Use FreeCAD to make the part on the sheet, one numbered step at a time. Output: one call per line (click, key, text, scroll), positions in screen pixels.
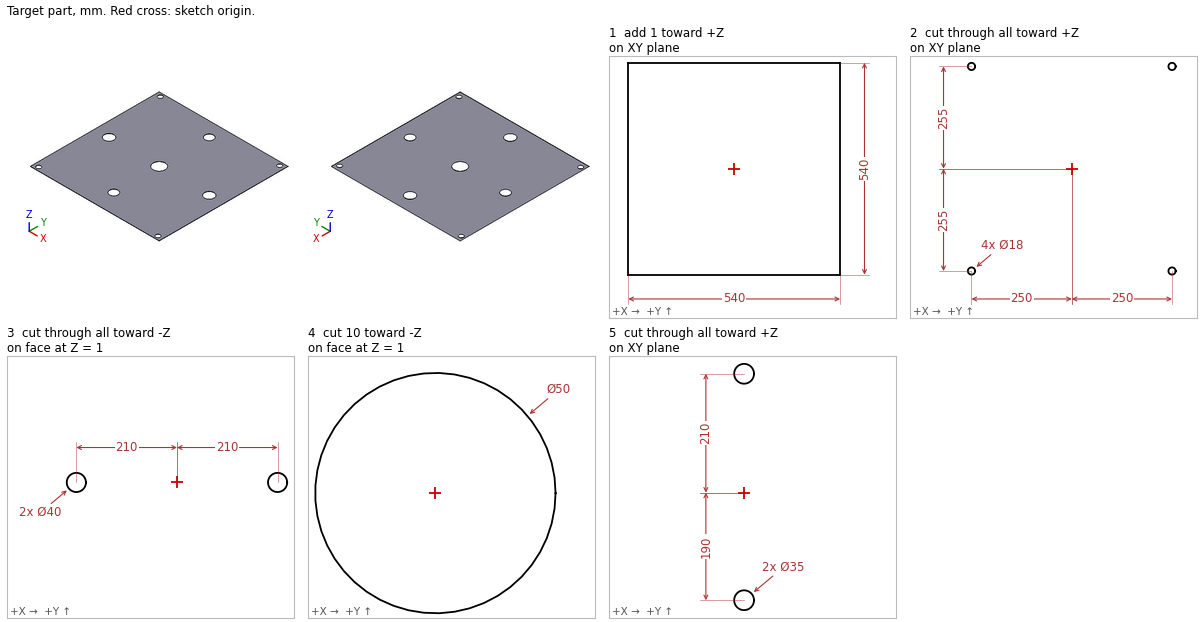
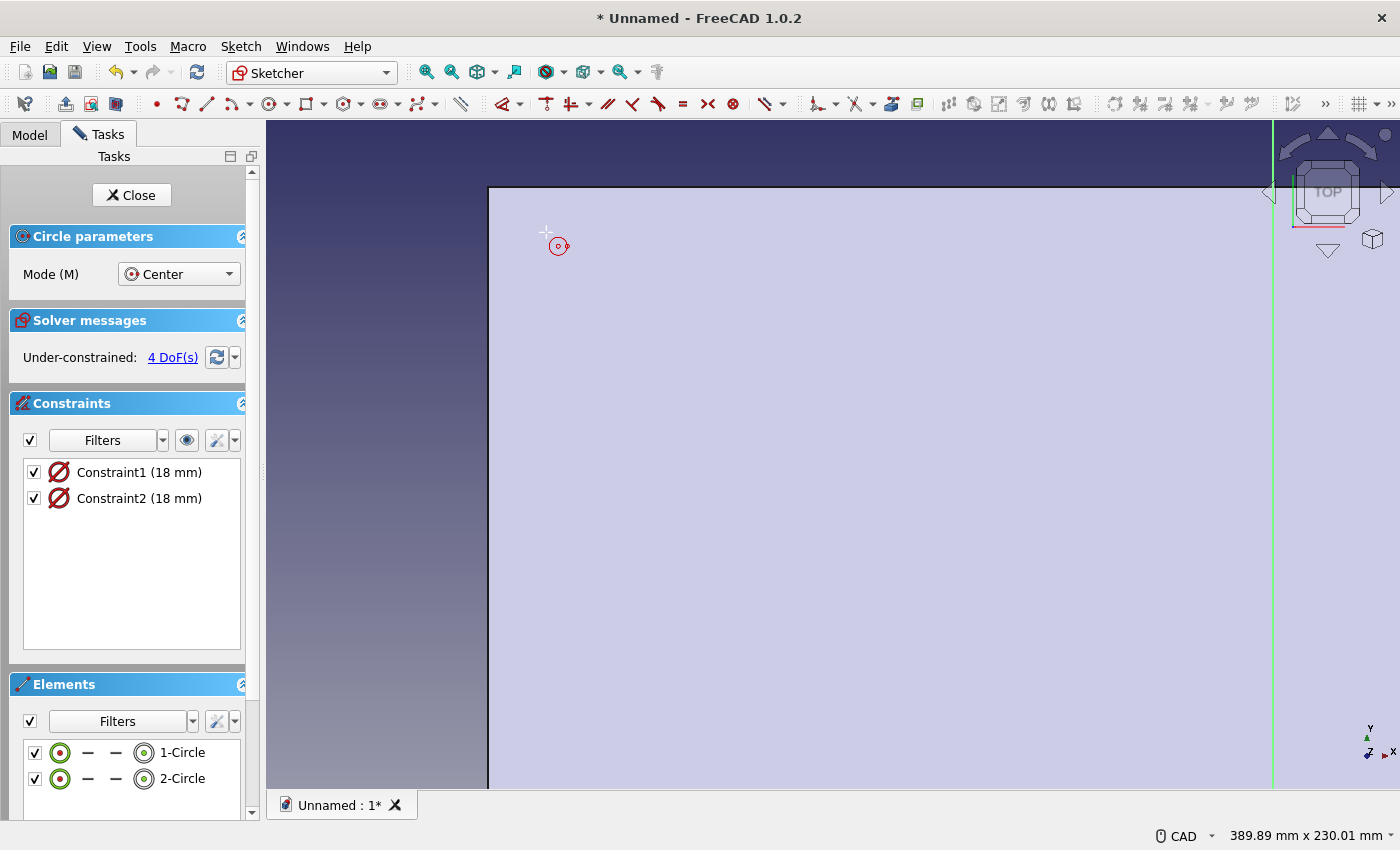
click(546, 231)
move(564, 212)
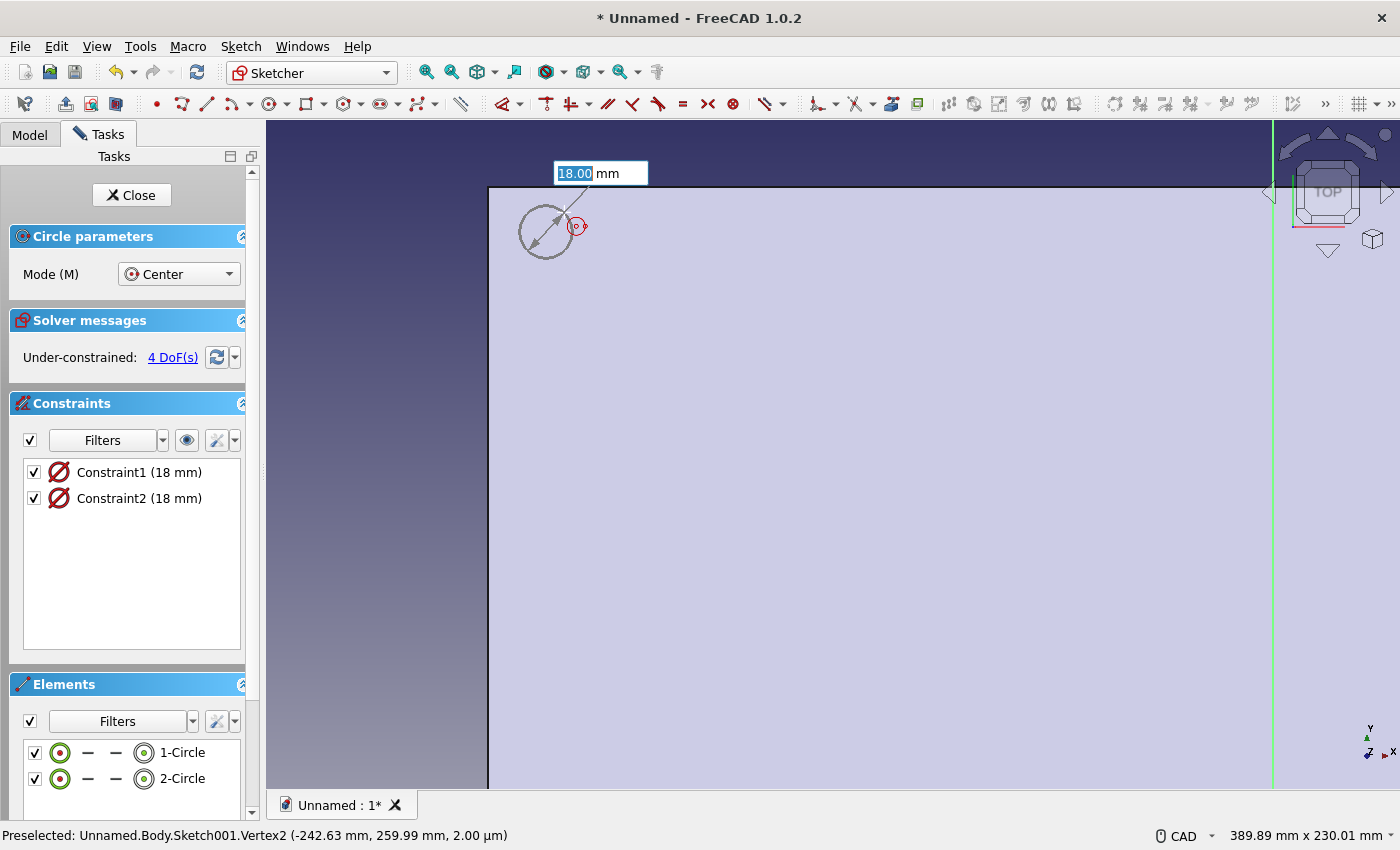
text(18)
key(Return)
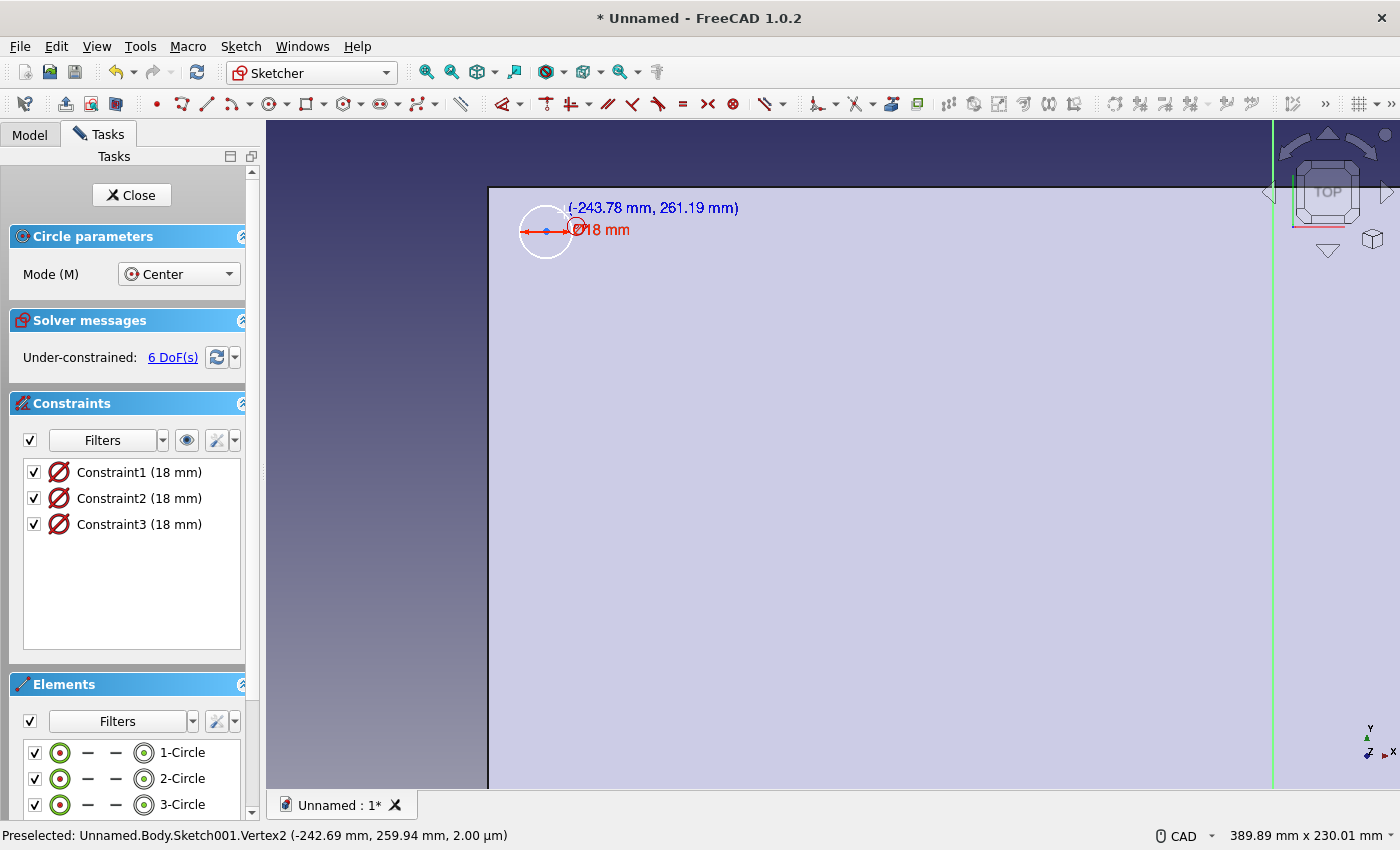
scroll(545, 231, down, 6)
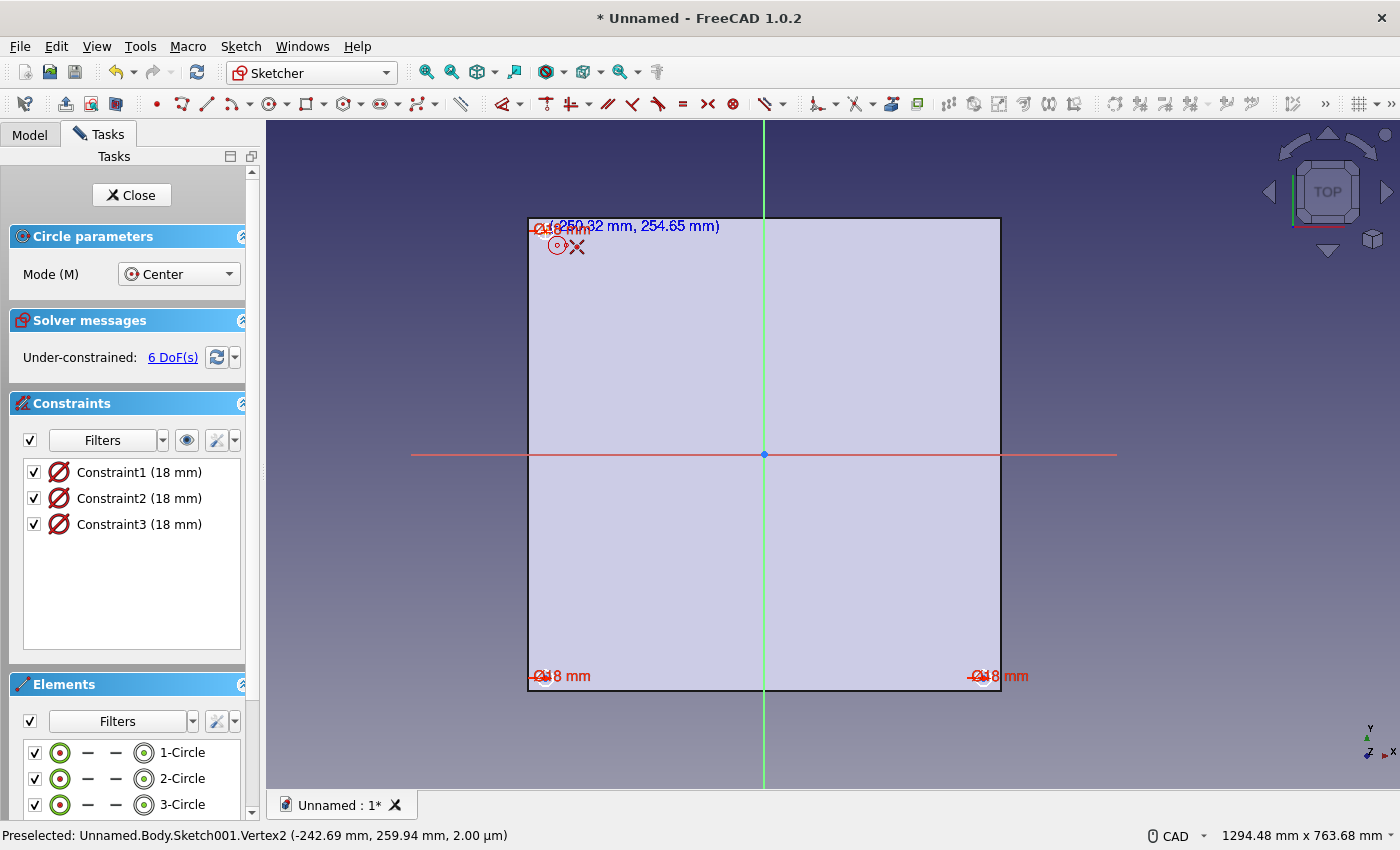
scroll(983, 231, up, 6)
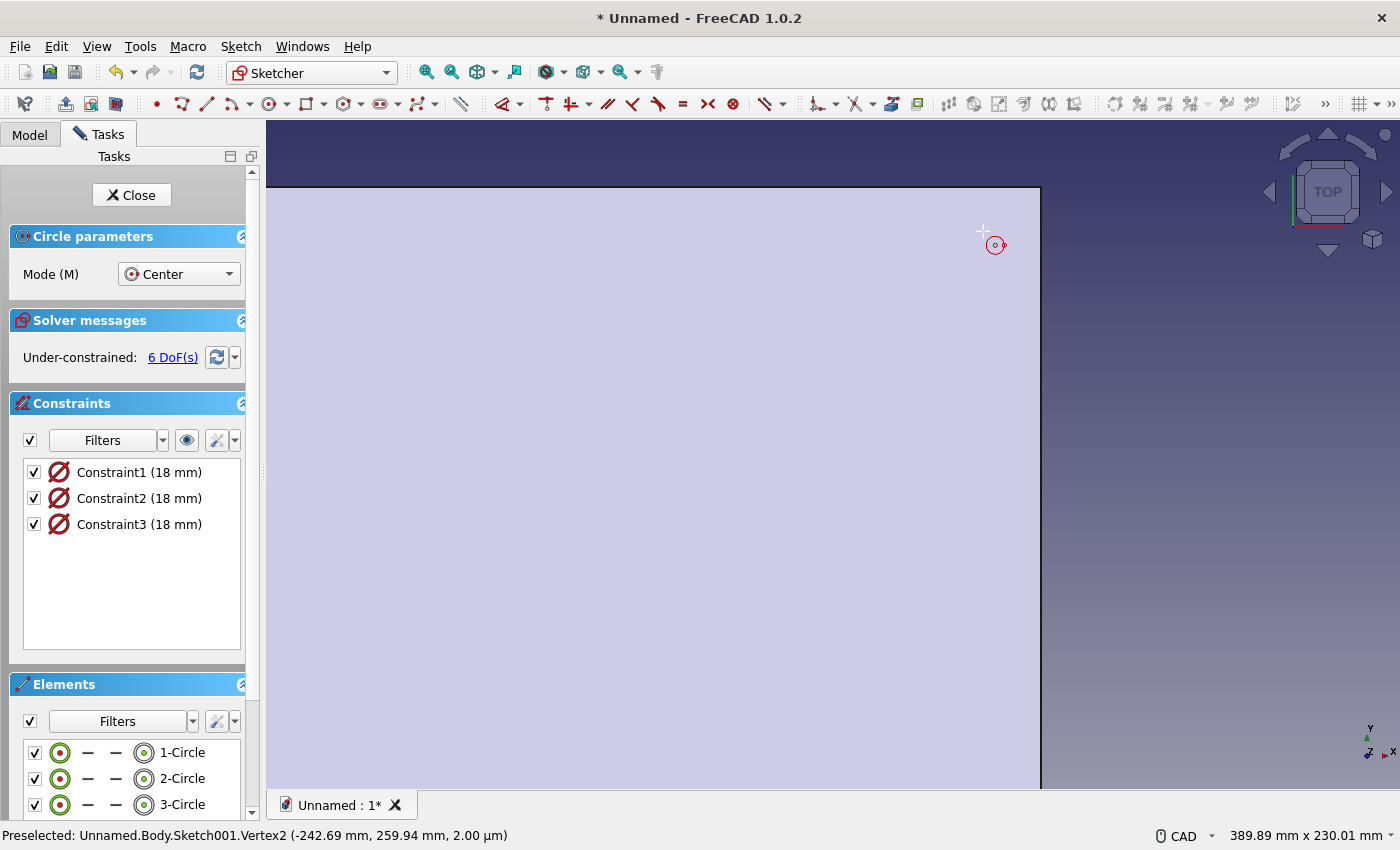
click(983, 231)
move(1002, 212)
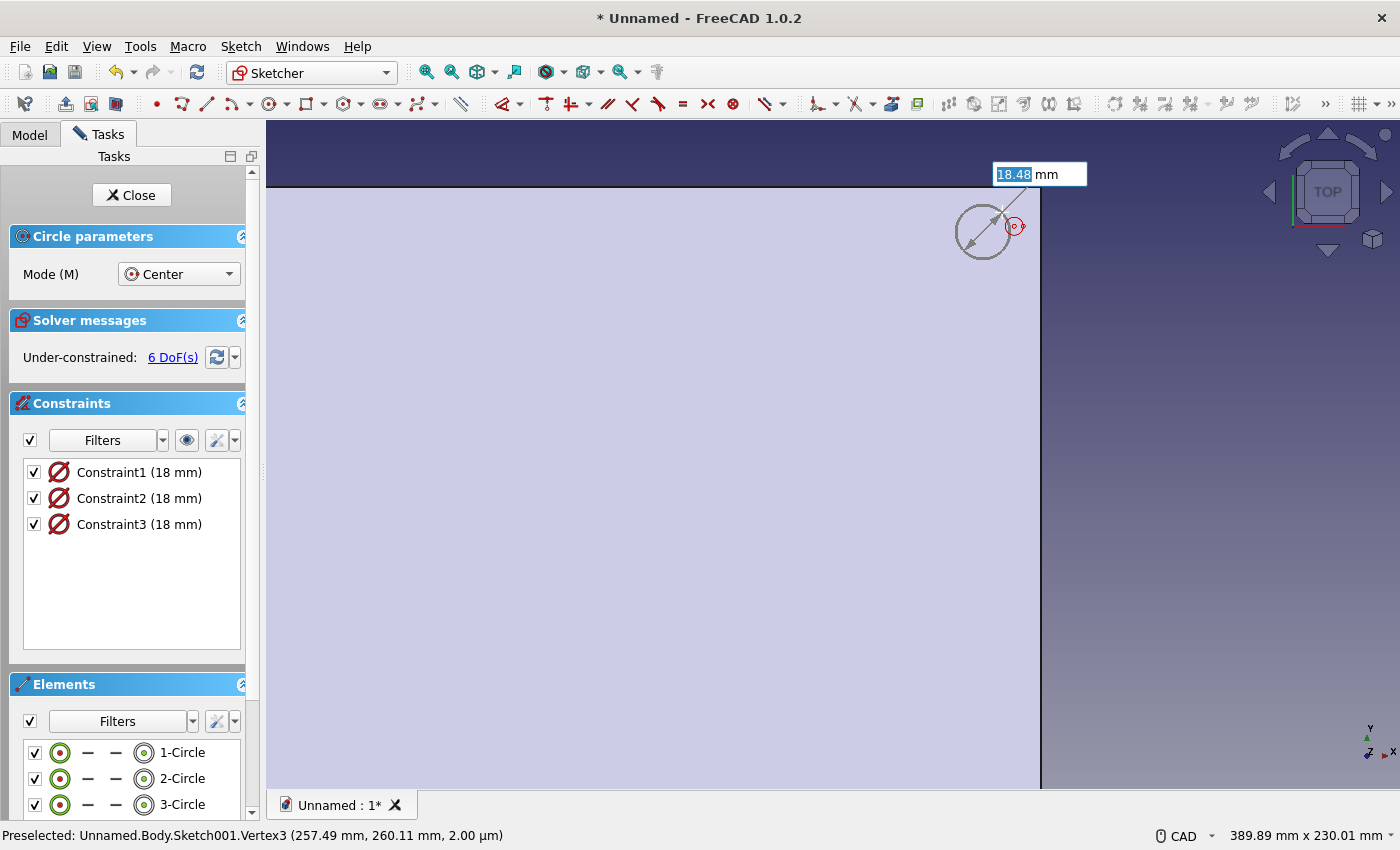
text(18)
key(Return)
key(Escape)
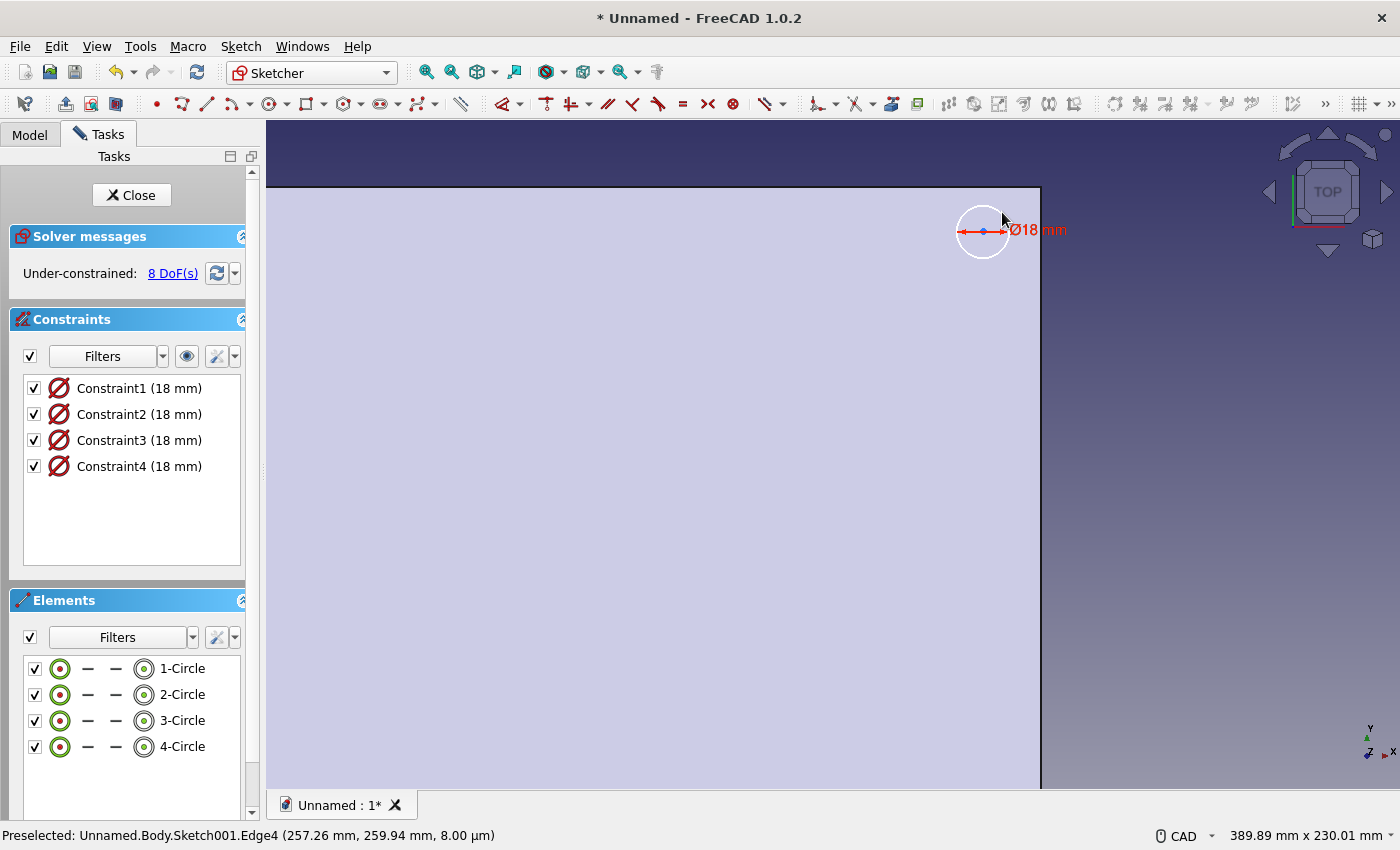
scroll(984, 231, down, 6)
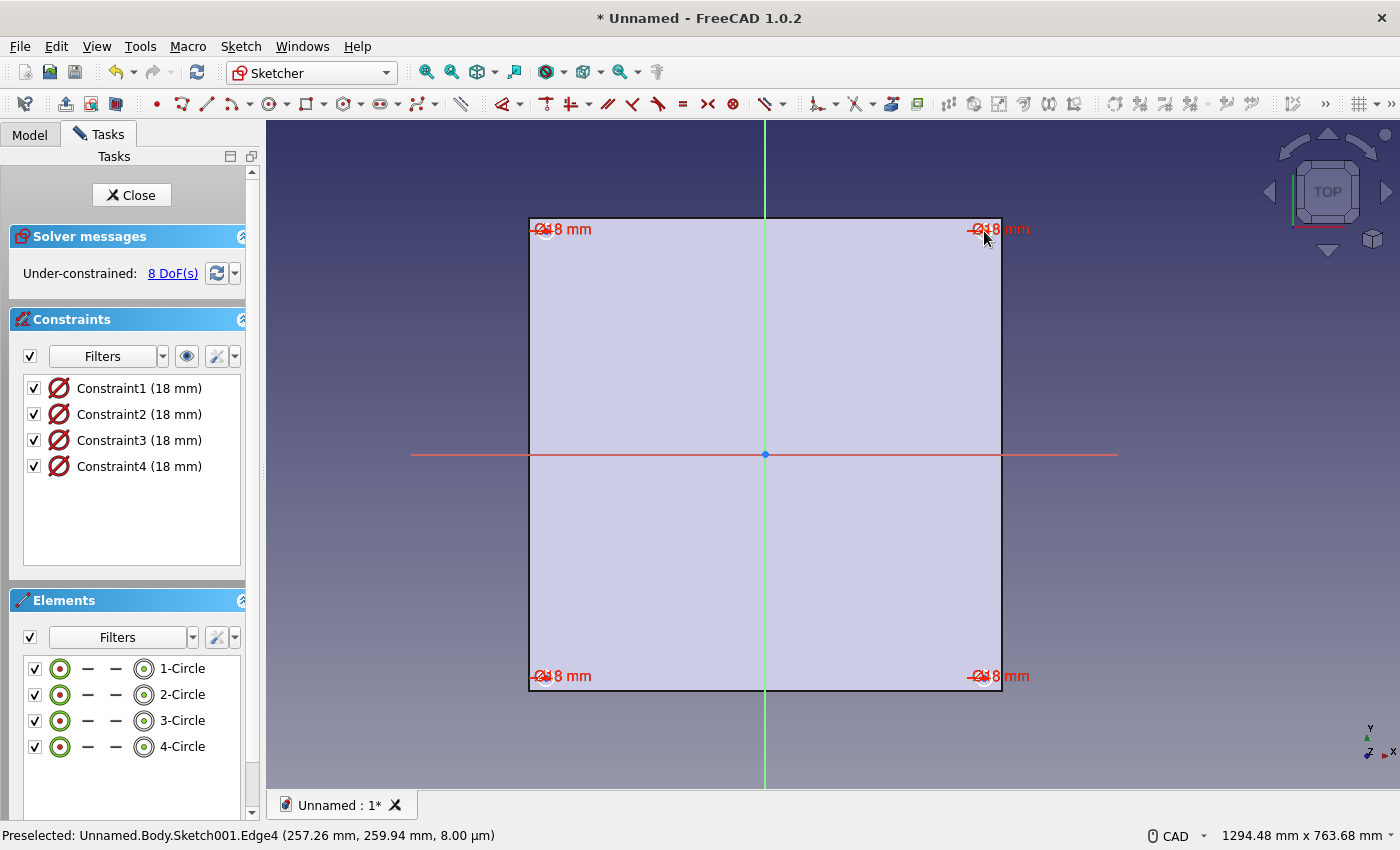
click(546, 678)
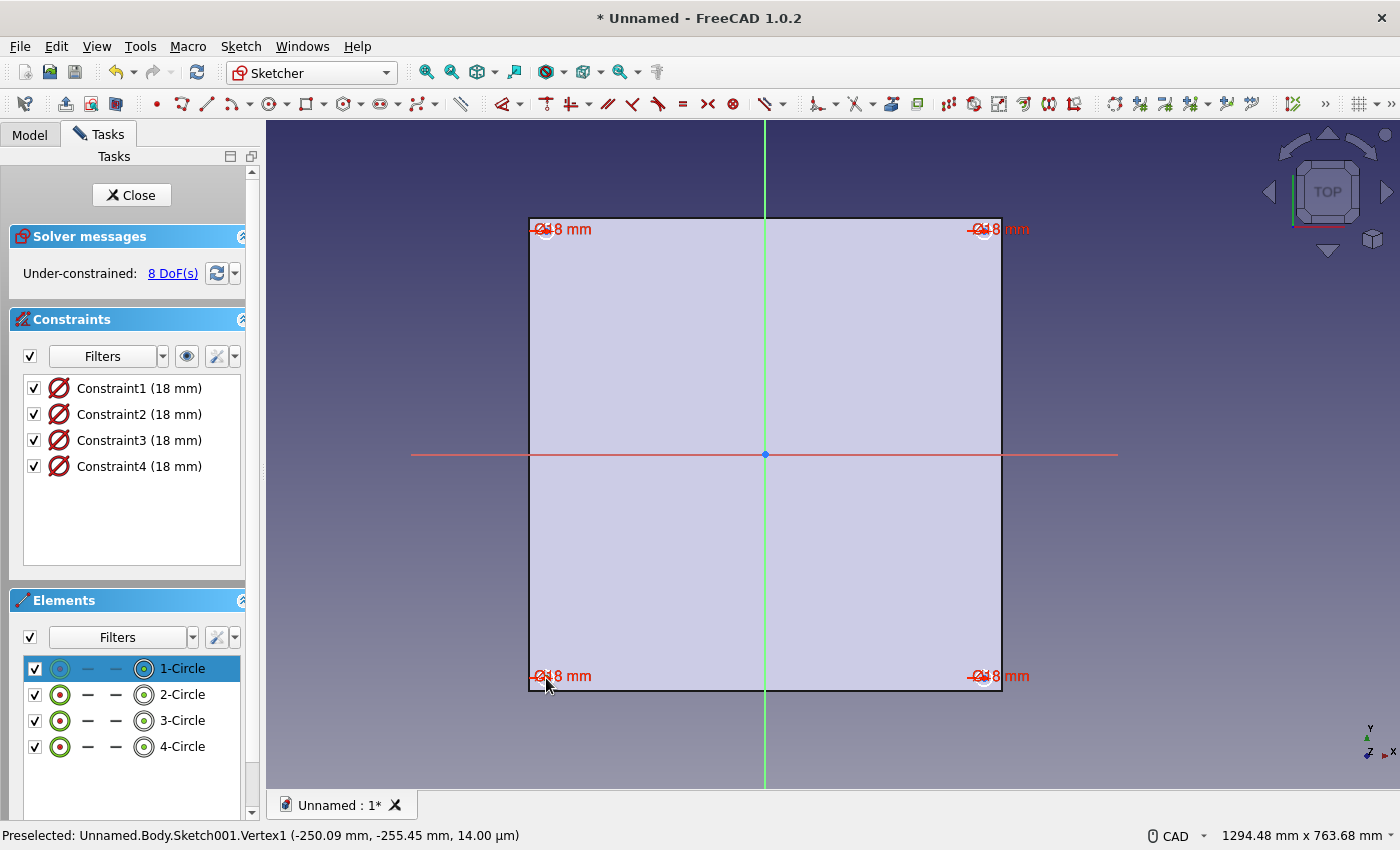
click(984, 678)